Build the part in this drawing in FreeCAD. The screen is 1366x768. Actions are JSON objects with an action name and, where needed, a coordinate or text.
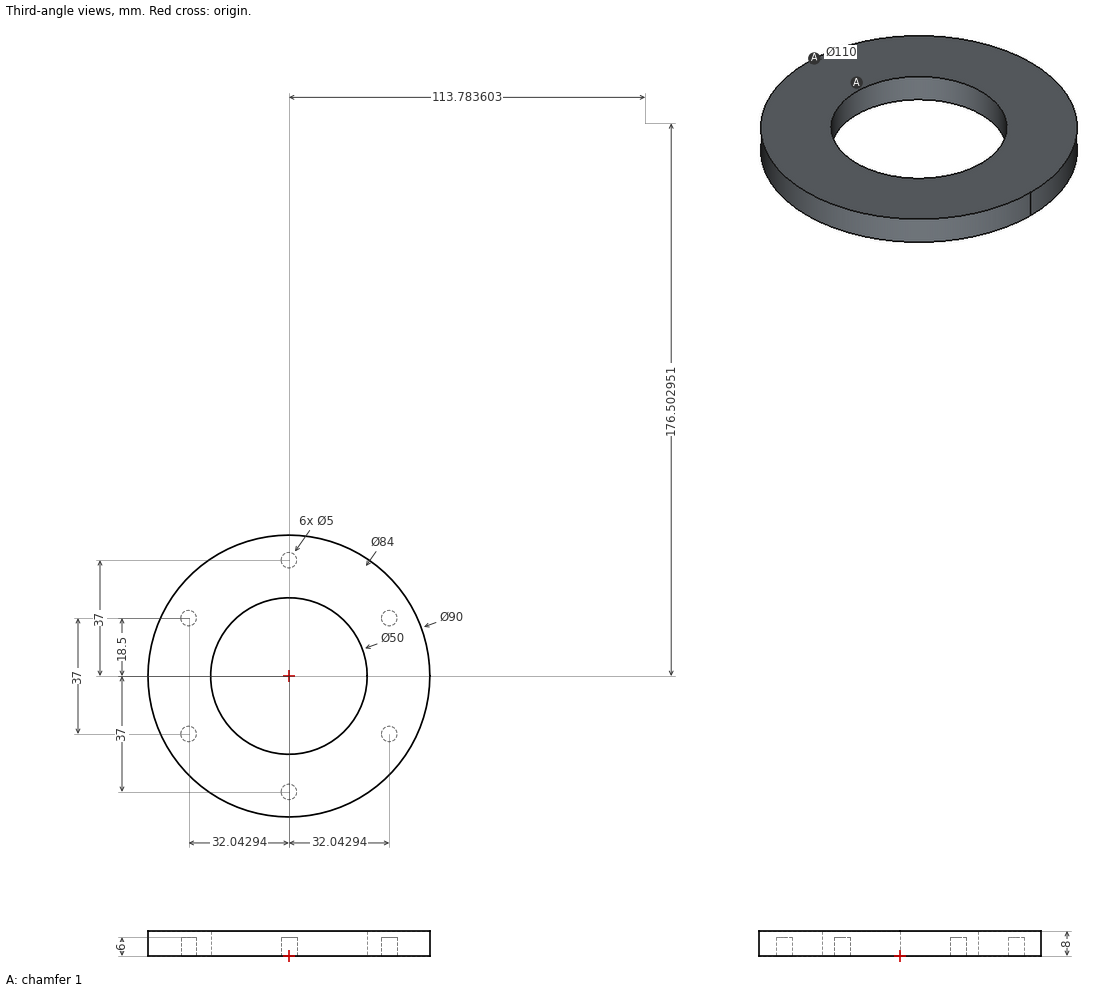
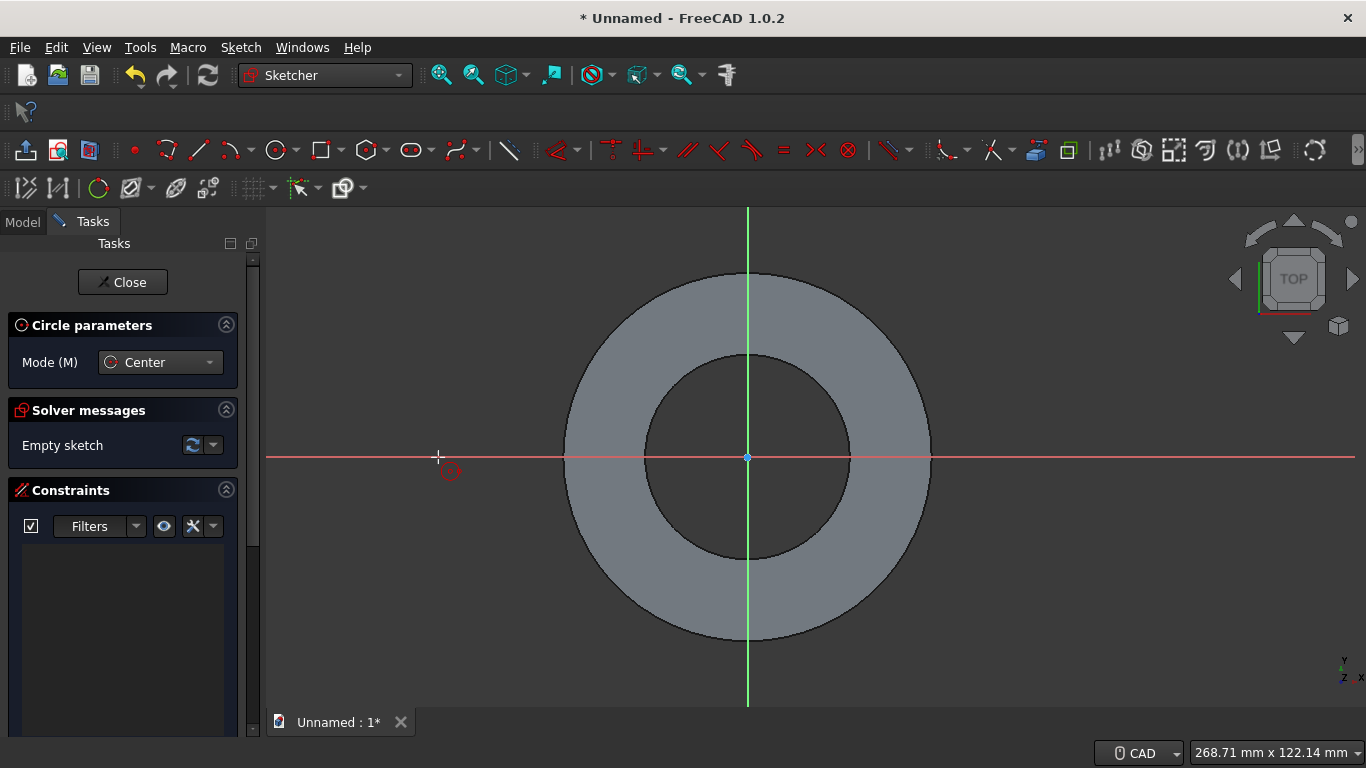
{"action": "left_click", "coordinate": [748, 457]}
{"action": "mouse_move", "coordinate": [869, 336]}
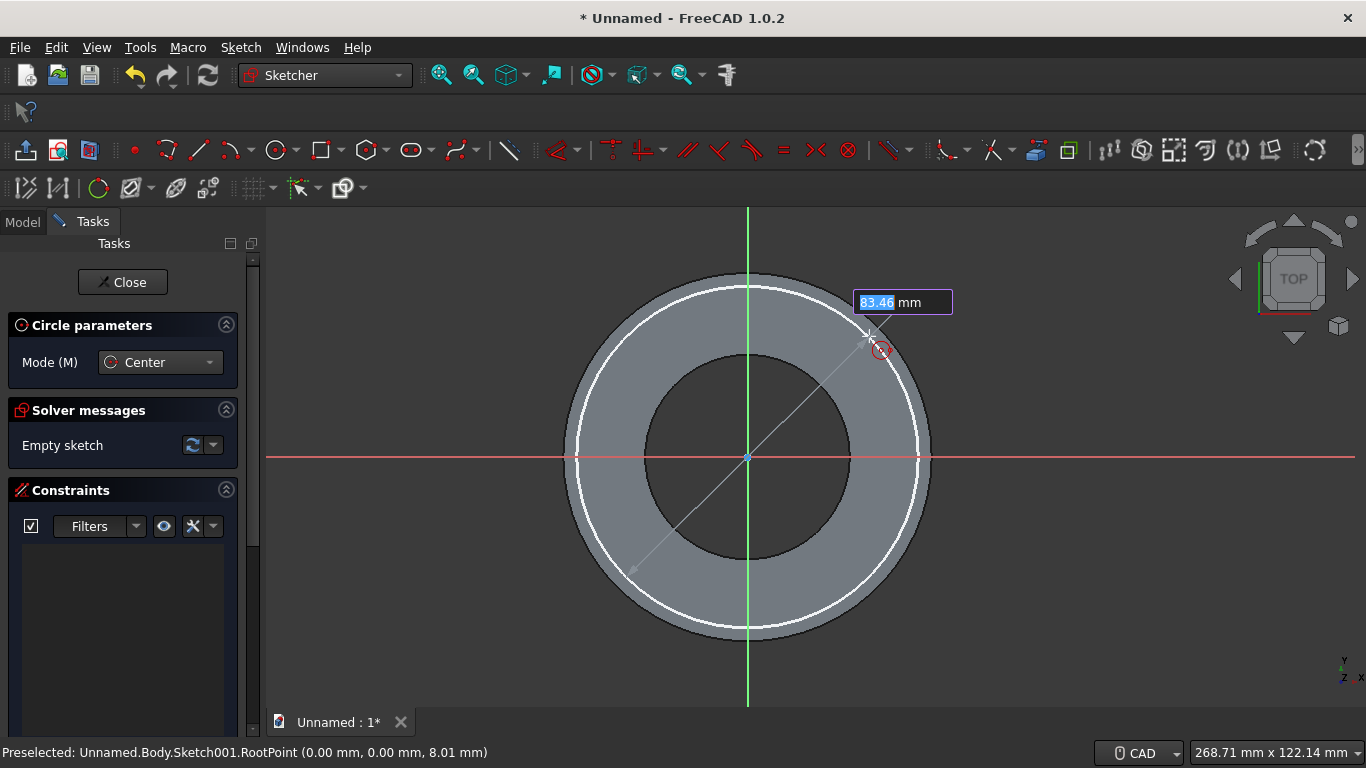
{"action": "type", "text": "84"}
{"action": "key", "text": "Return"}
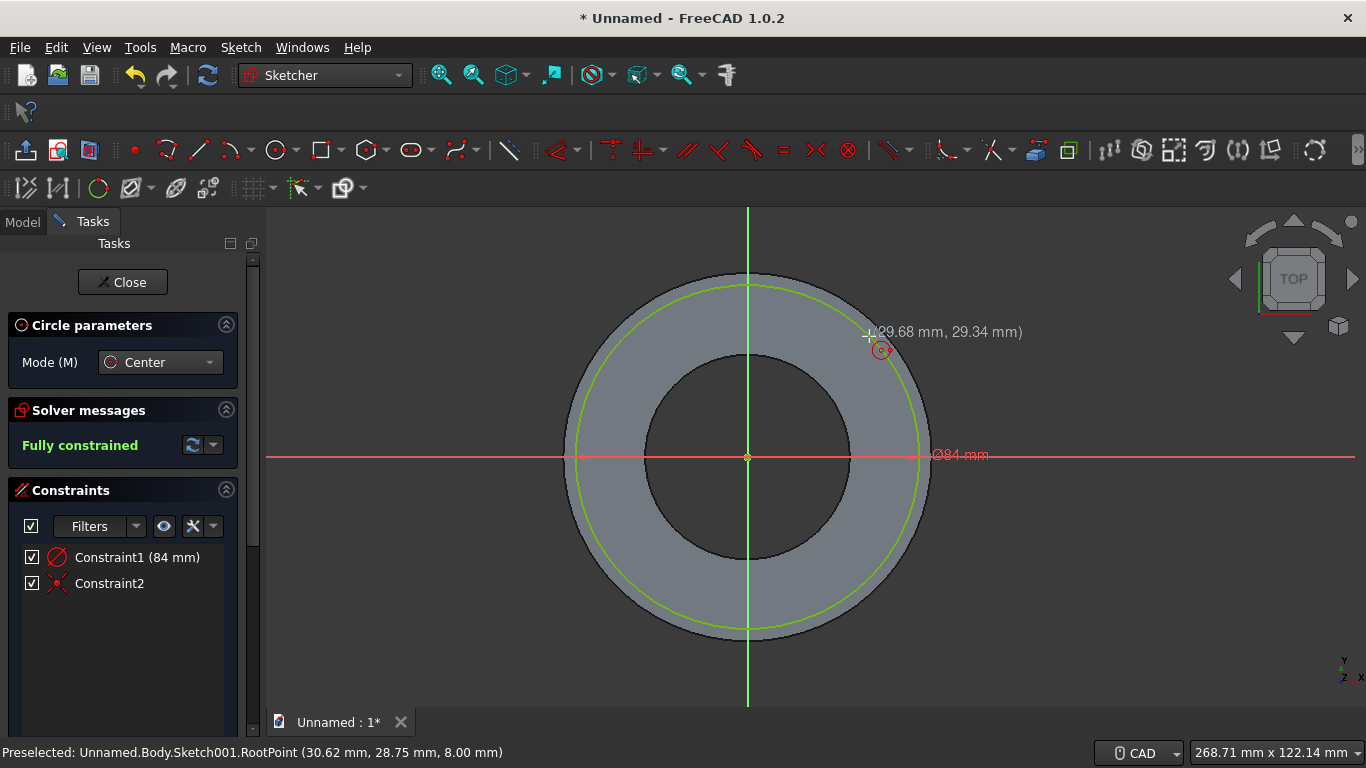
{"action": "left_click", "coordinate": [748, 457]}
{"action": "mouse_move", "coordinate": [820, 385]}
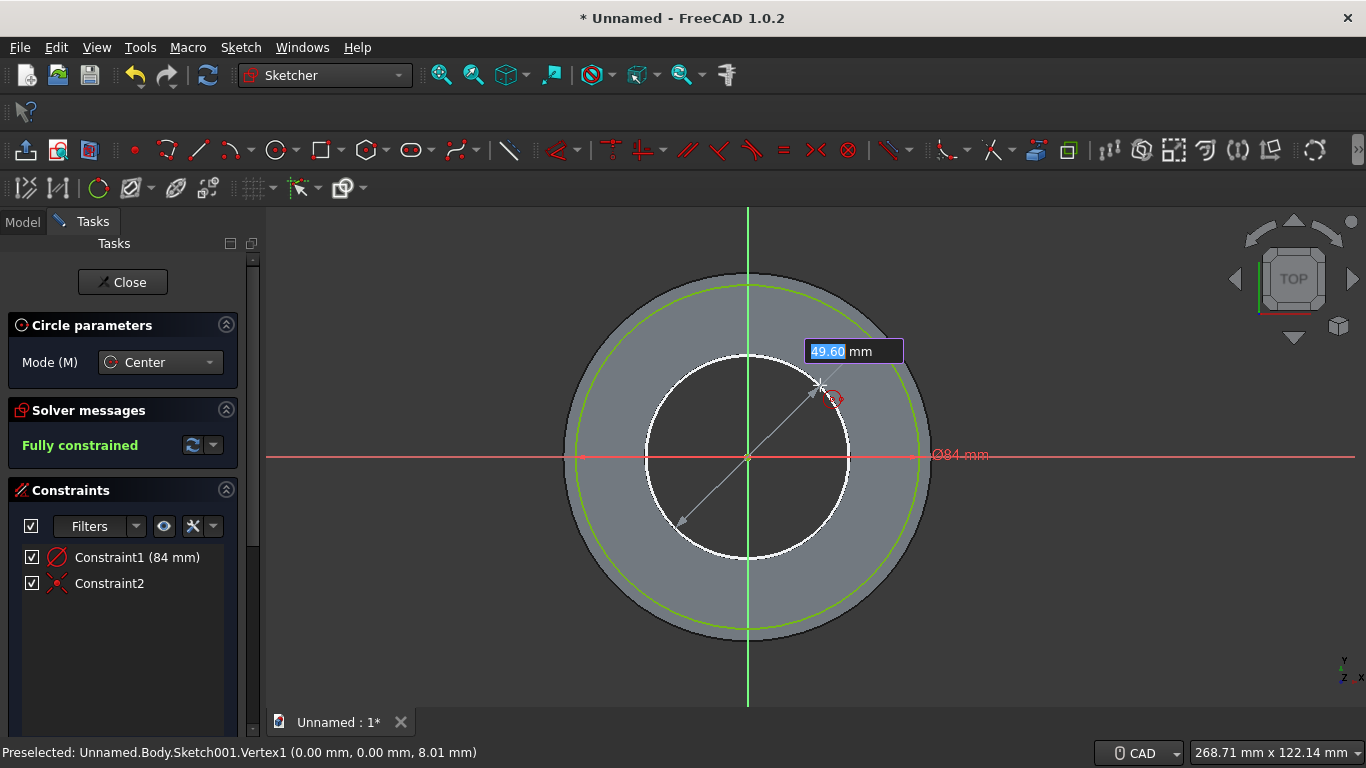
{"action": "type", "text": "50"}
{"action": "key", "text": "Return"}
{"action": "key", "text": "Escape"}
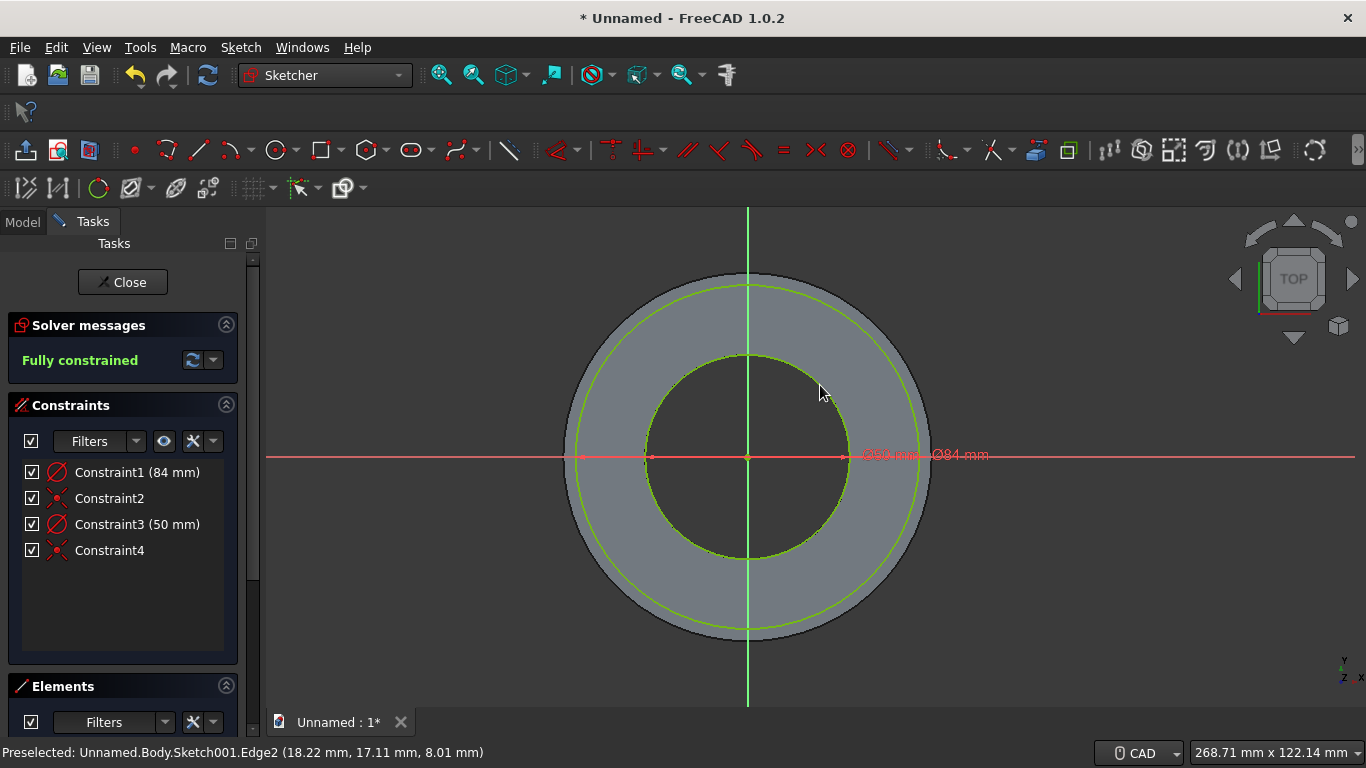
{"action": "left_click", "coordinate": [123, 282]}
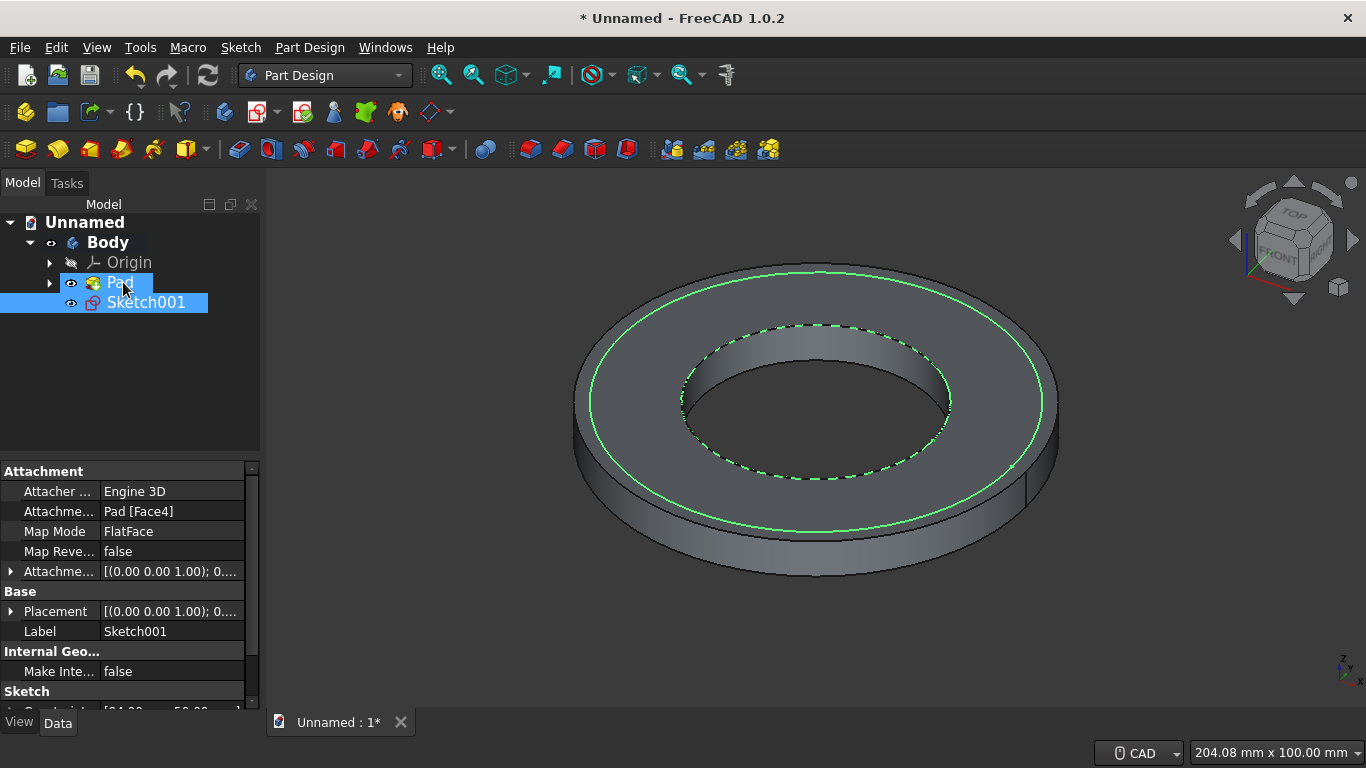
{"action": "left_click", "coordinate": [26, 150]}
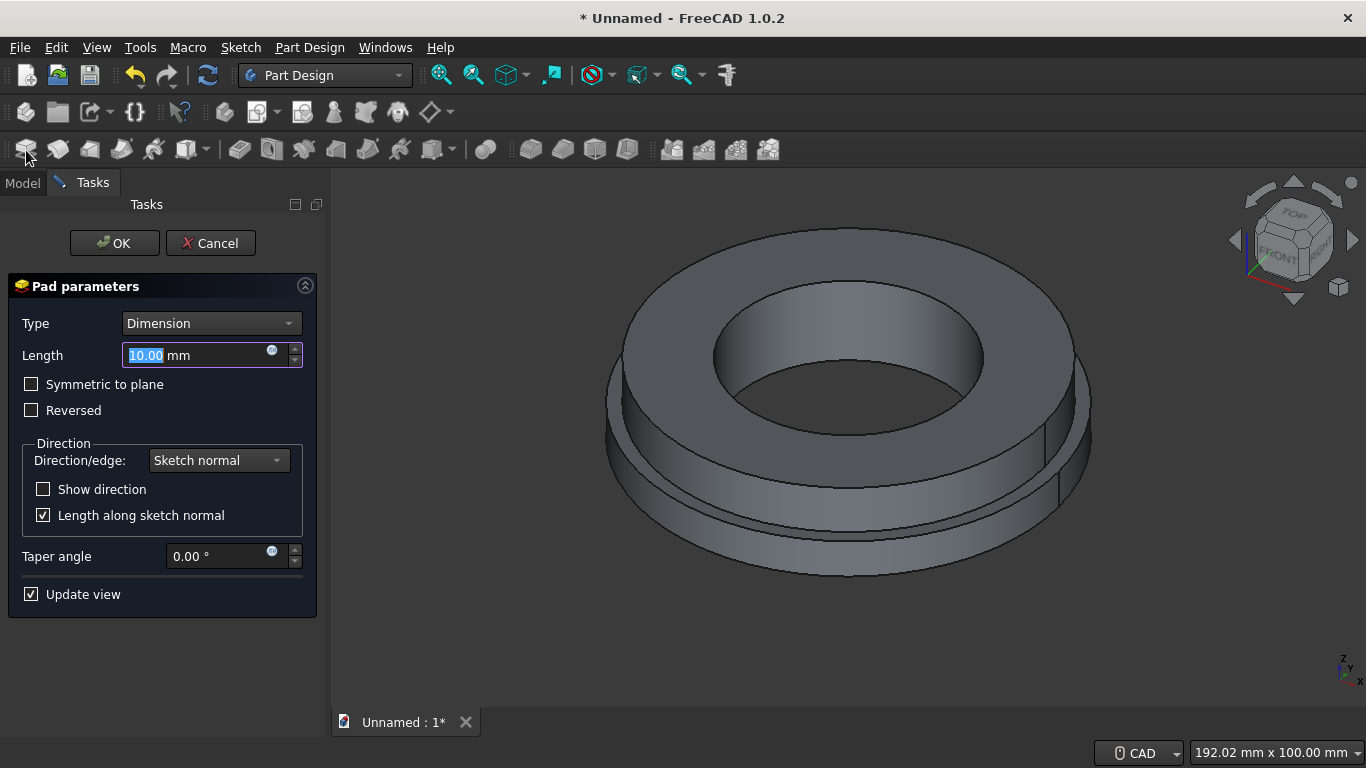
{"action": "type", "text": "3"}
{"action": "key", "text": "Tab"}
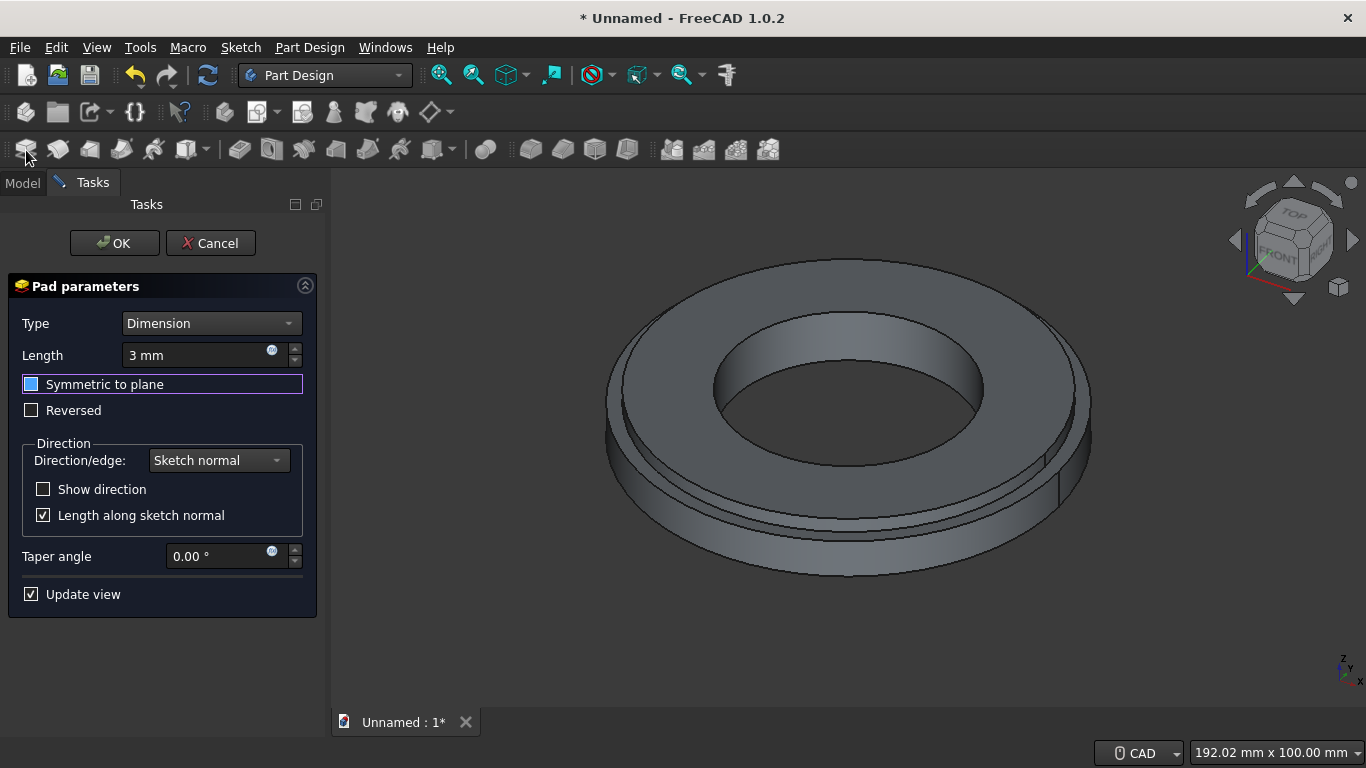
{"action": "left_click", "coordinate": [115, 243]}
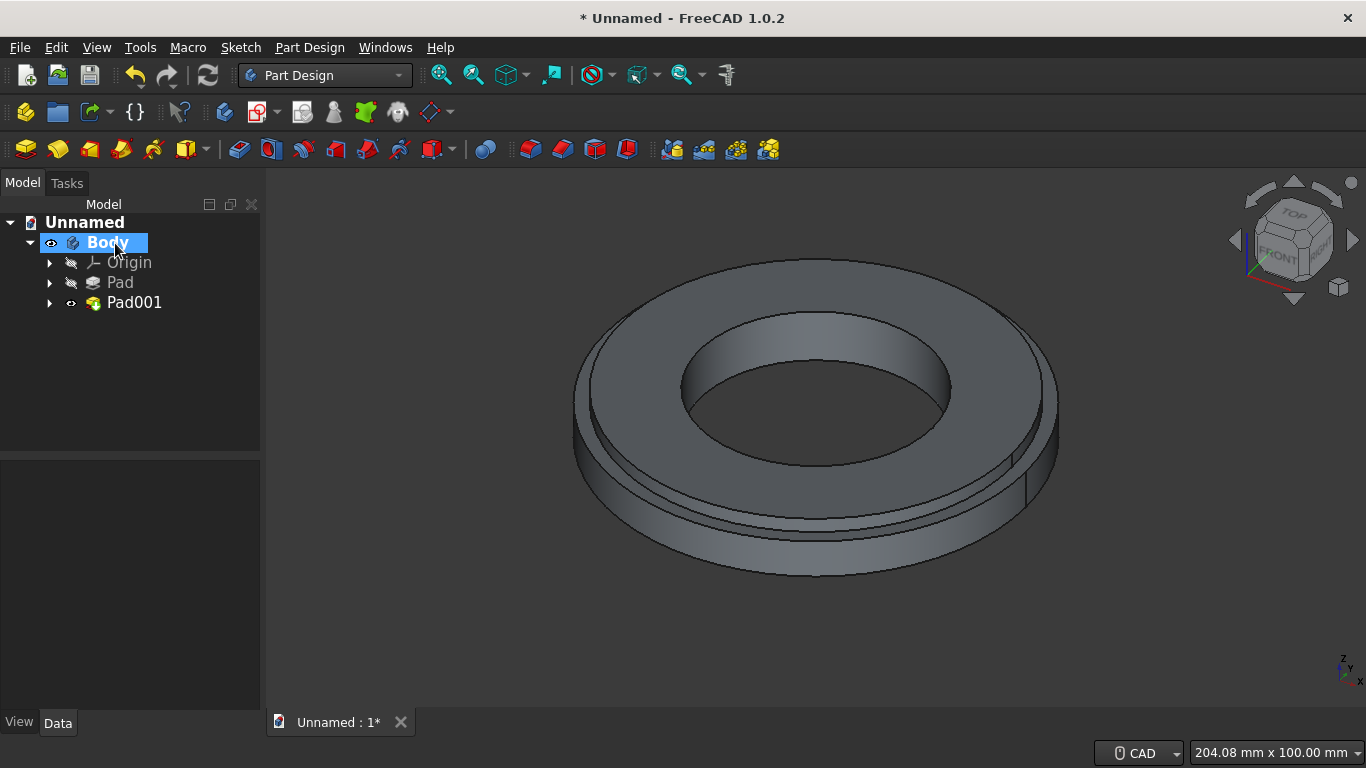
{"action": "key", "text": "5"}